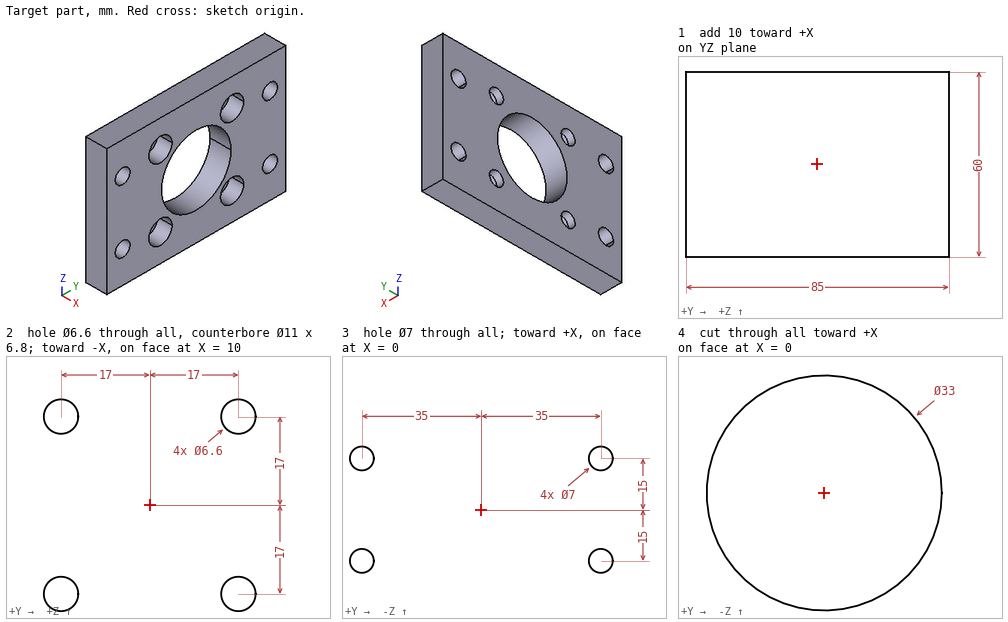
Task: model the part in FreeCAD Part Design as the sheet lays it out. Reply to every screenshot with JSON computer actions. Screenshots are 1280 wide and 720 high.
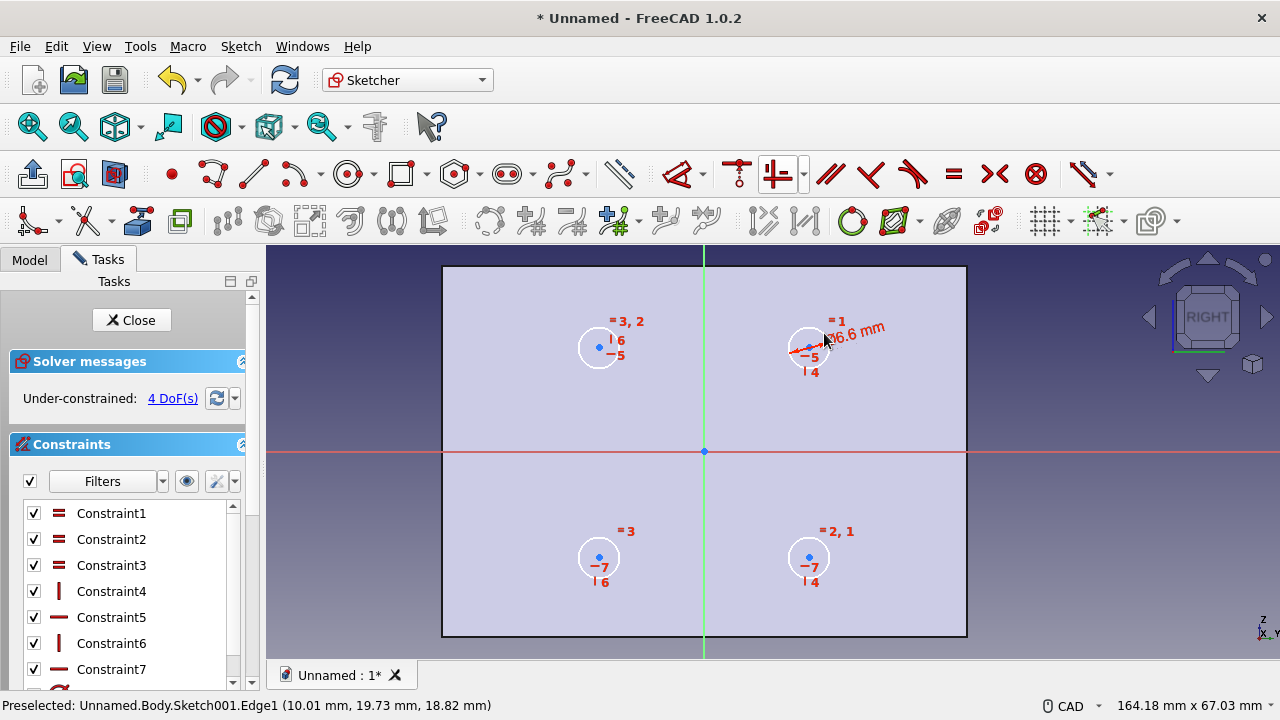
{"action": "left_click", "coordinate": [809, 348]}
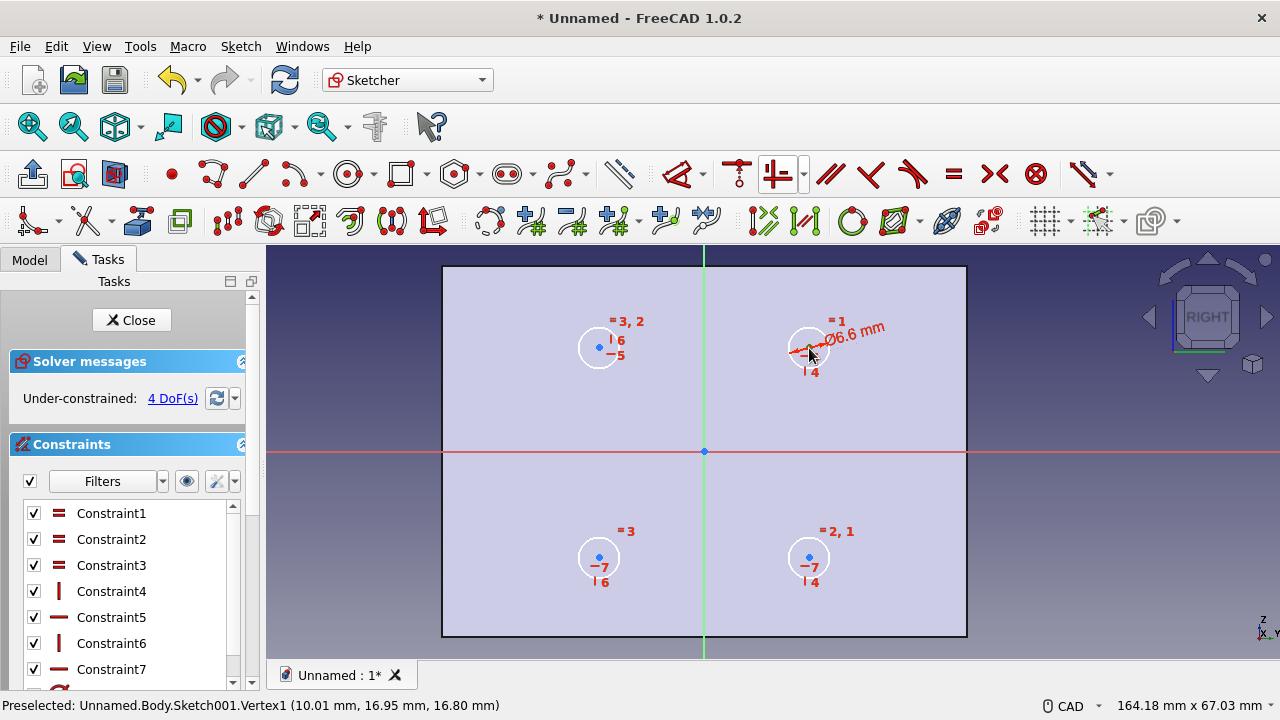
{"action": "left_click", "coordinate": [702, 174]}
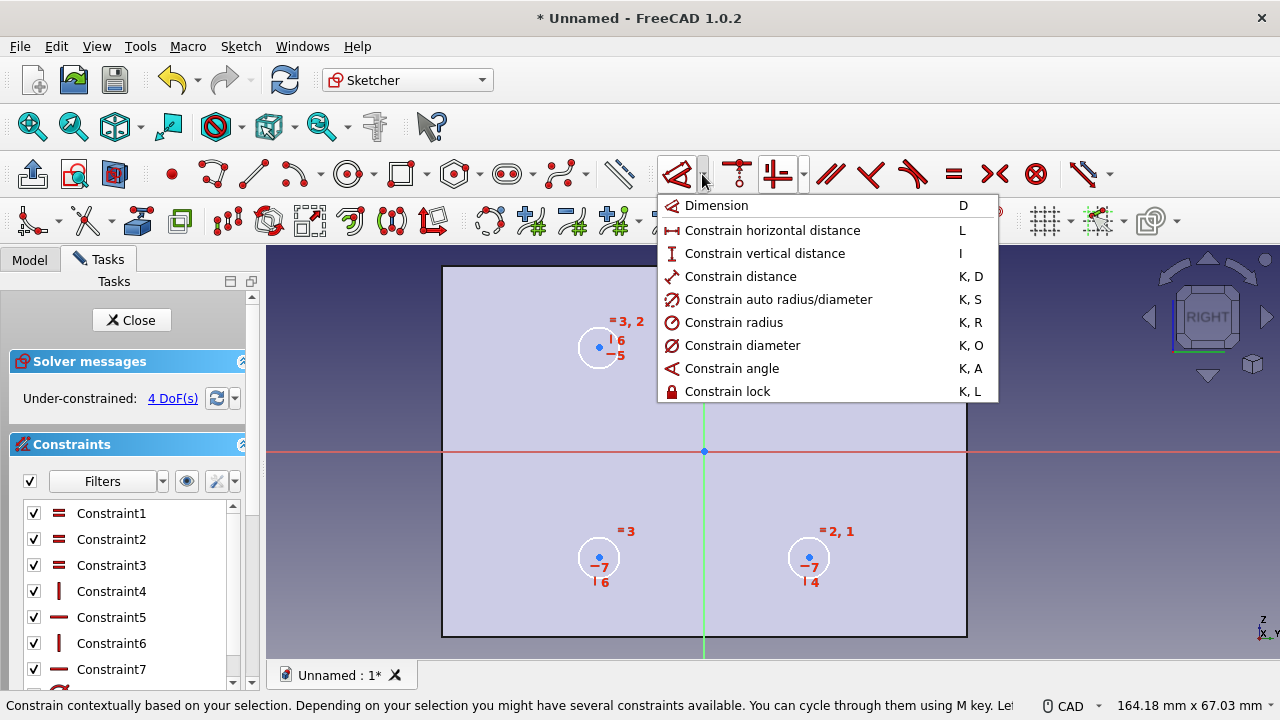
{"action": "left_click", "coordinate": [828, 230]}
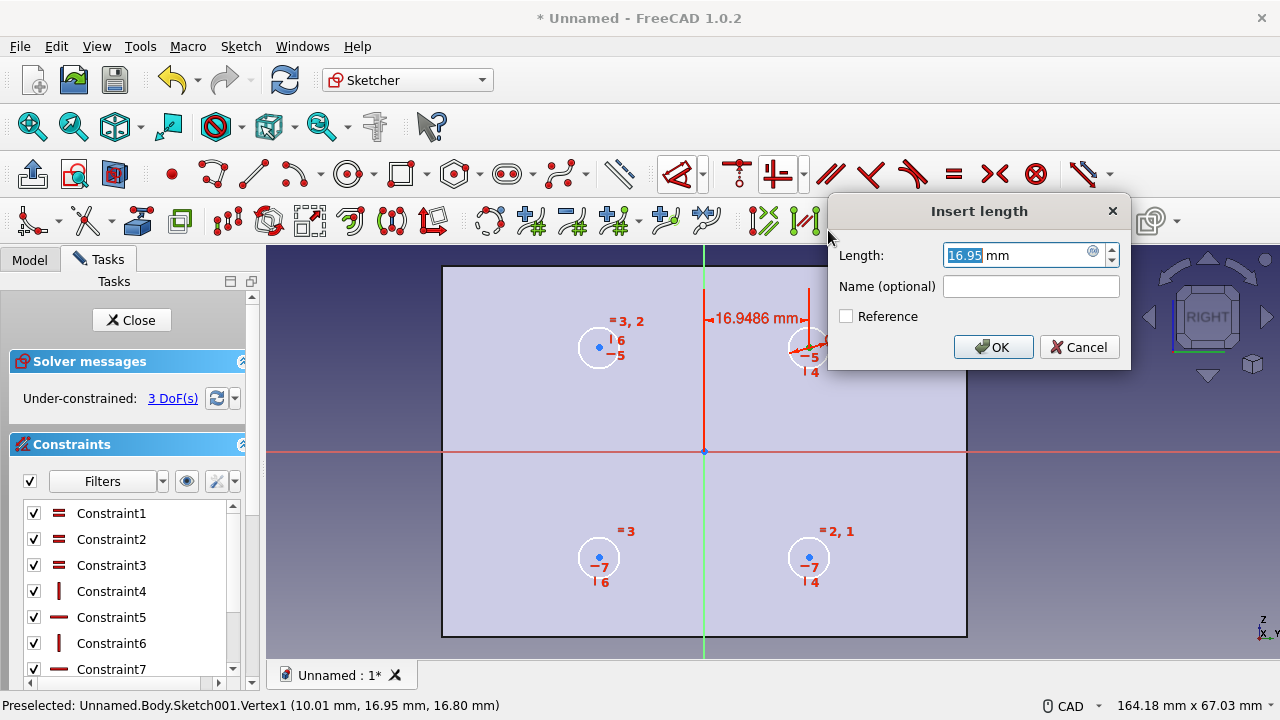
{"action": "type", "text": "17"}
{"action": "key", "text": "Return"}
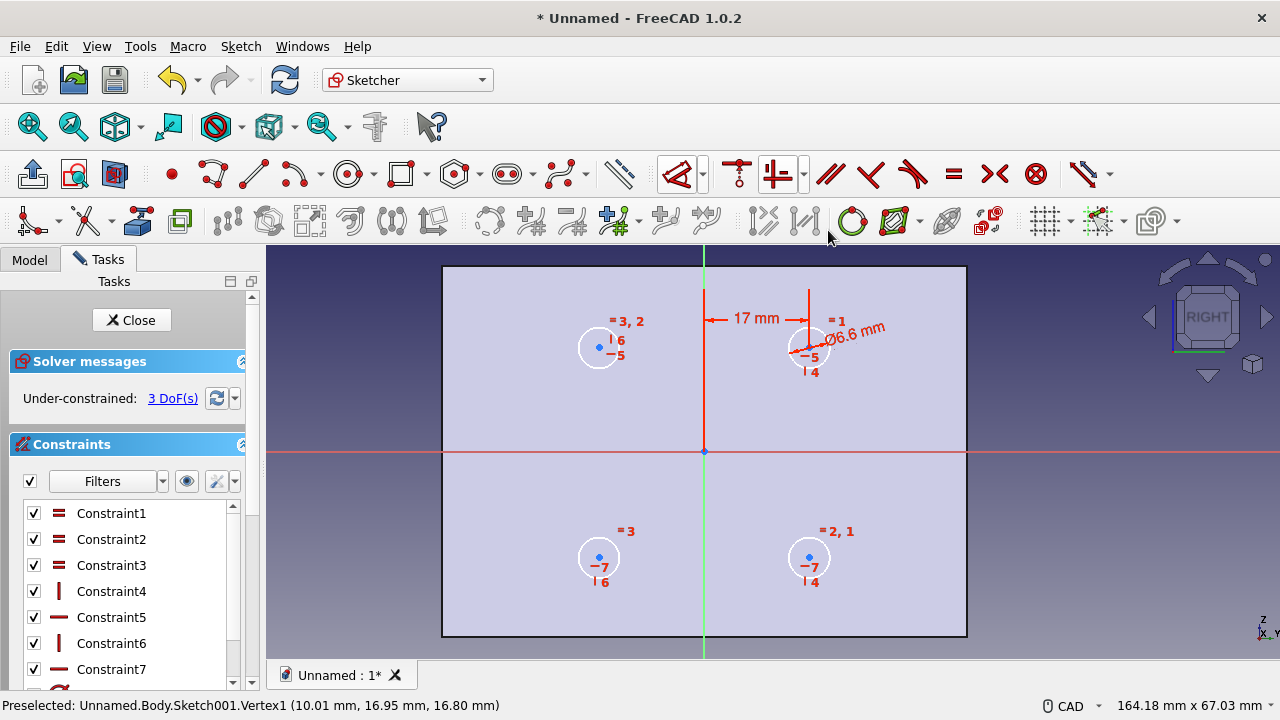
{"action": "left_click", "coordinate": [809, 348]}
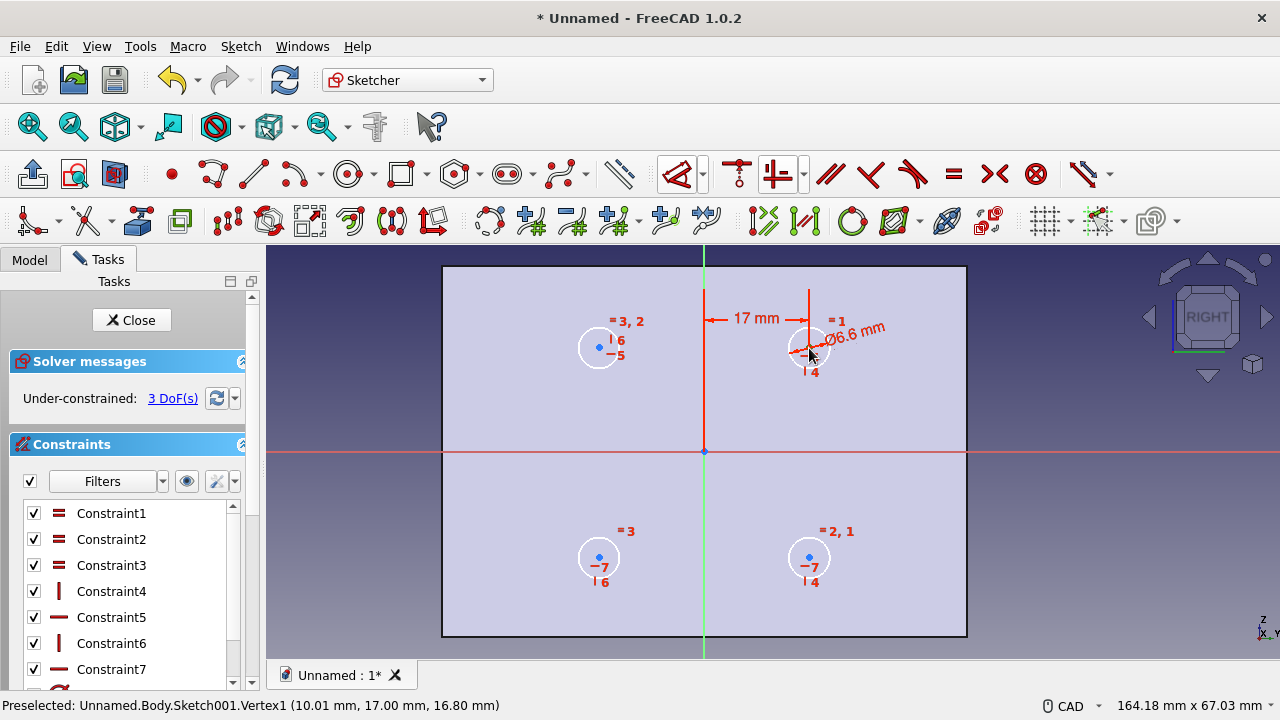
{"action": "key", "text": "i"}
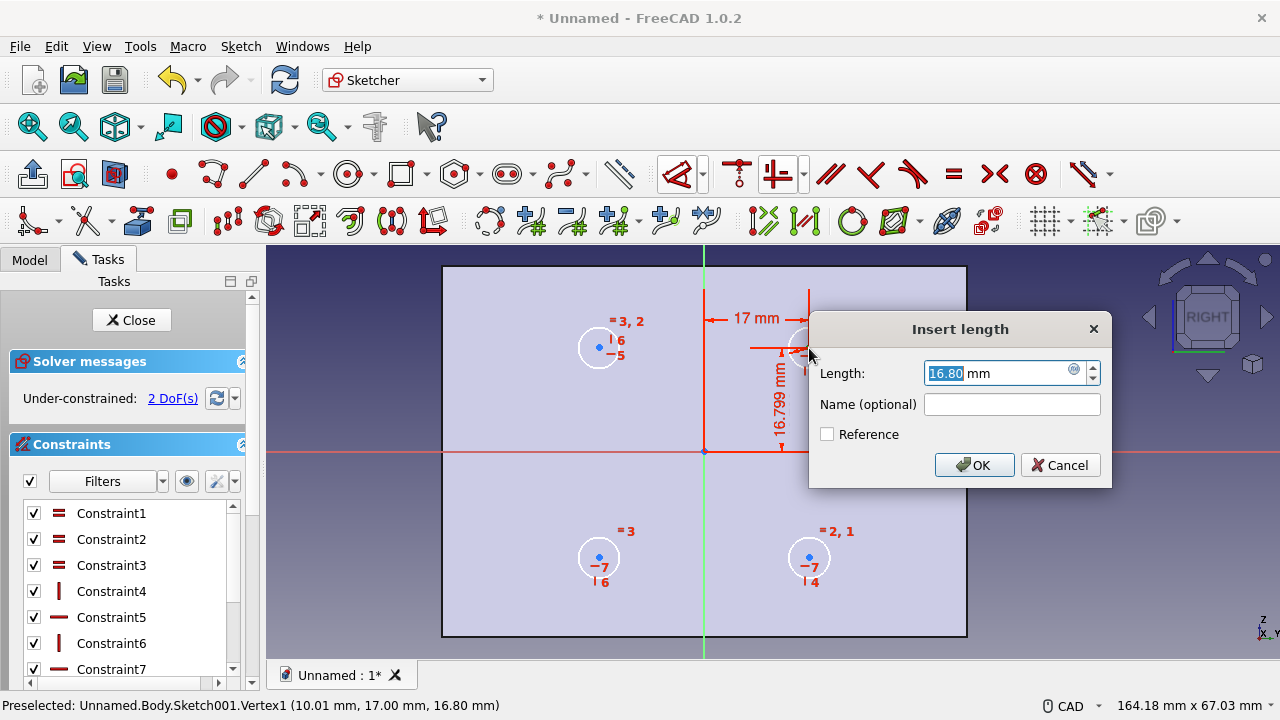
{"action": "type", "text": "17"}
{"action": "key", "text": "Return"}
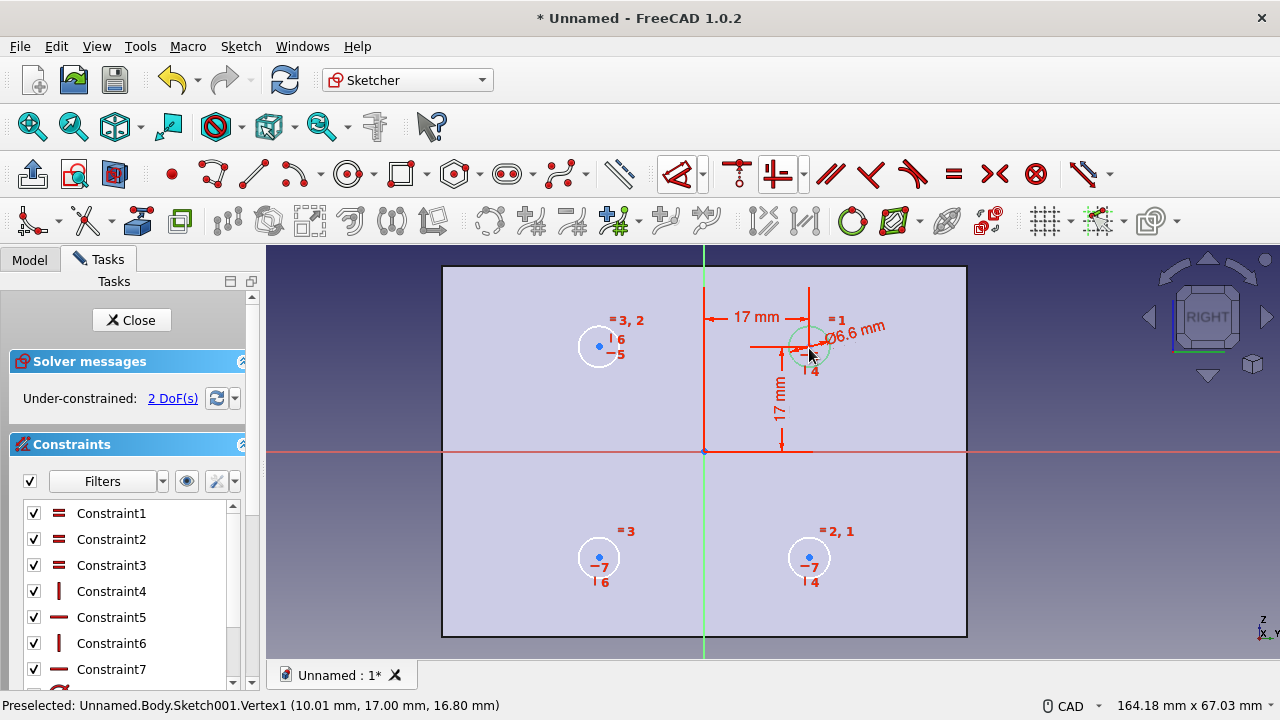
{"action": "left_click", "coordinate": [809, 558]}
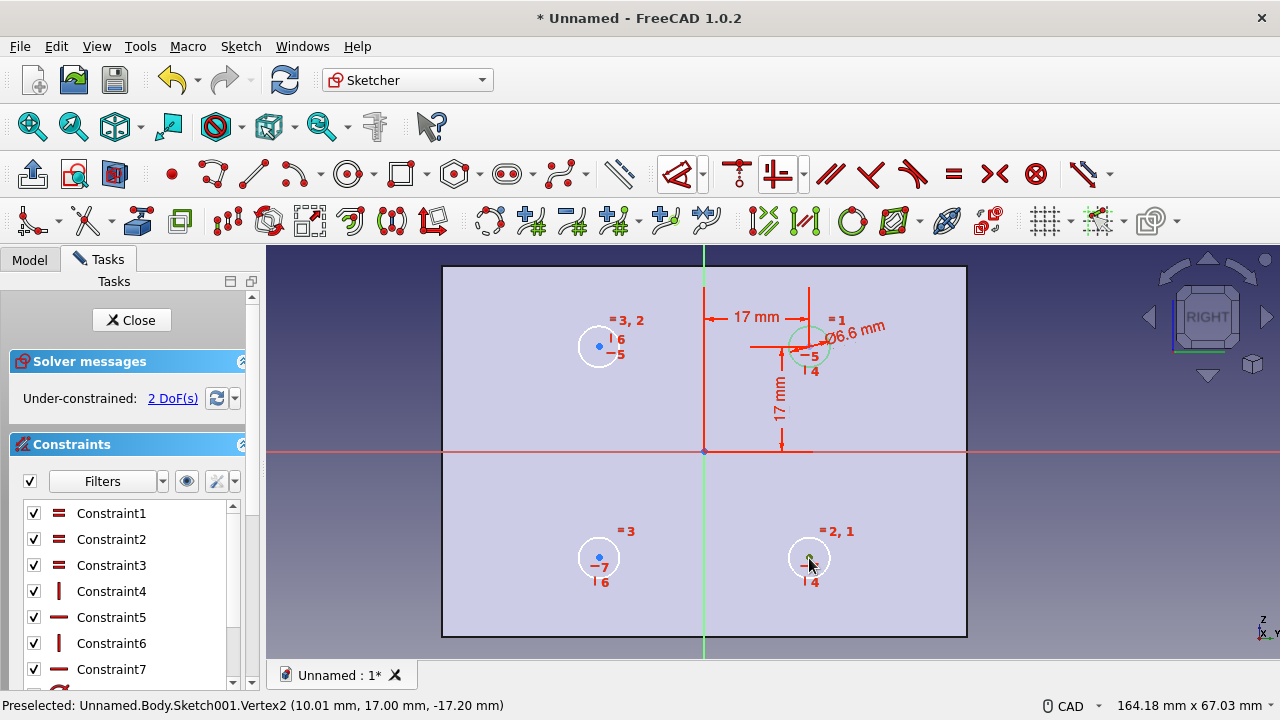
{"action": "left_click", "coordinate": [702, 174]}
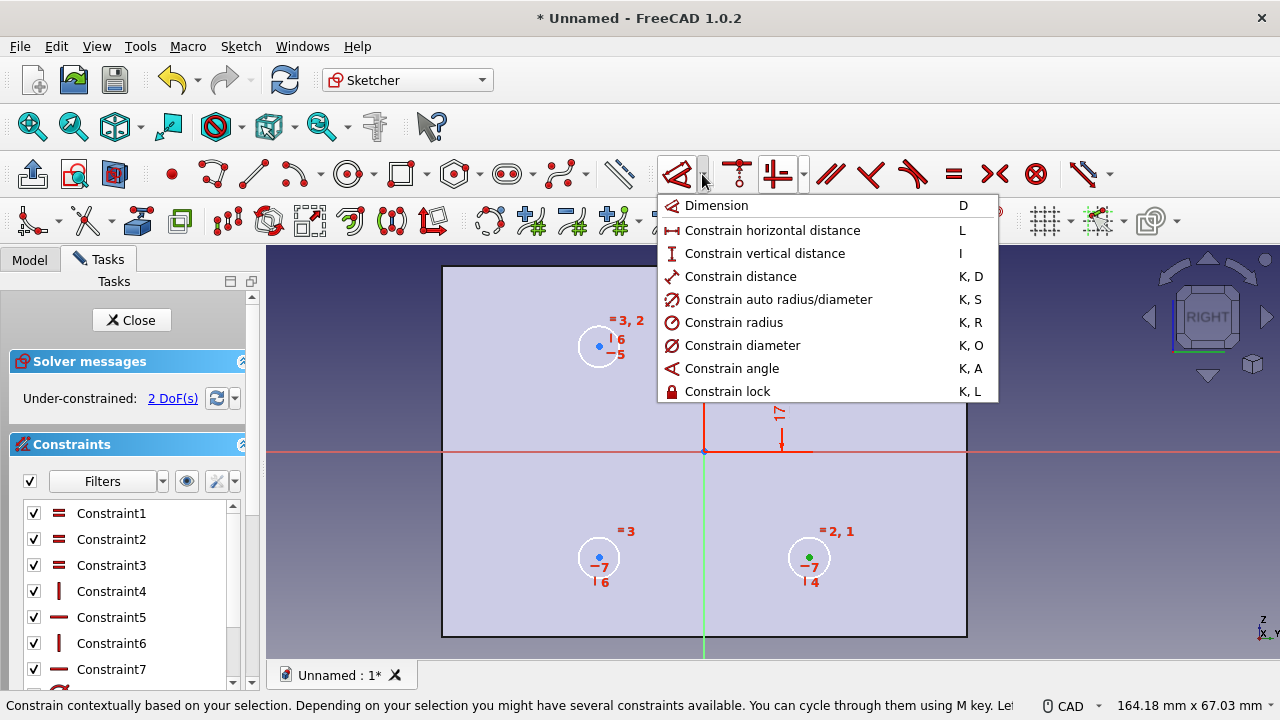
{"action": "left_click", "coordinate": [828, 254]}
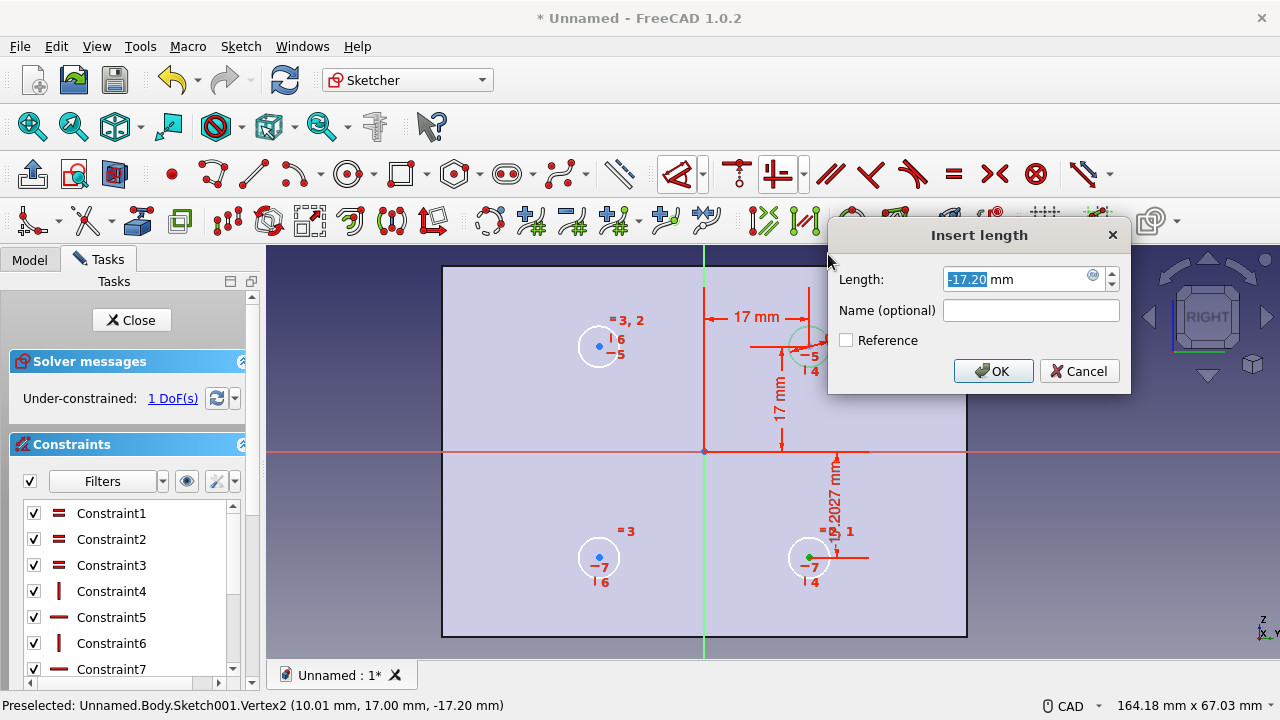
{"action": "type", "text": "-17"}
{"action": "key", "text": "Return"}